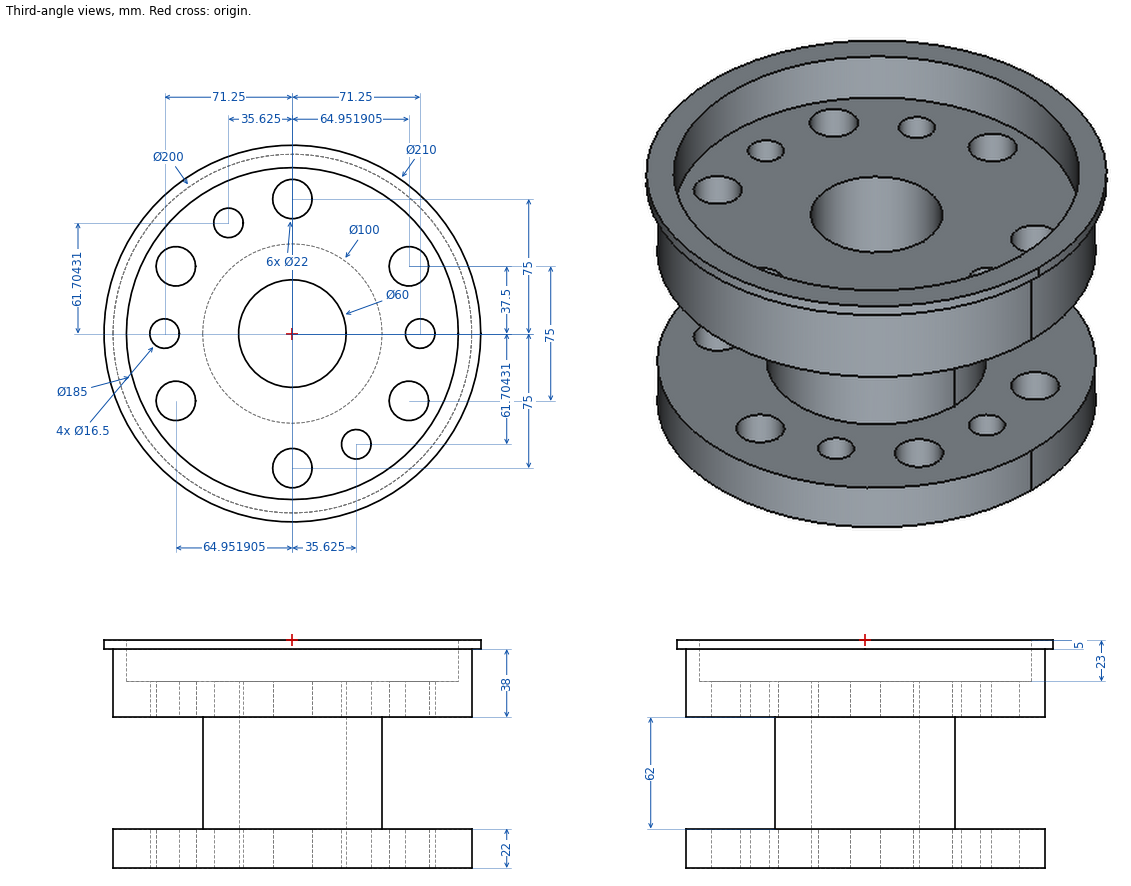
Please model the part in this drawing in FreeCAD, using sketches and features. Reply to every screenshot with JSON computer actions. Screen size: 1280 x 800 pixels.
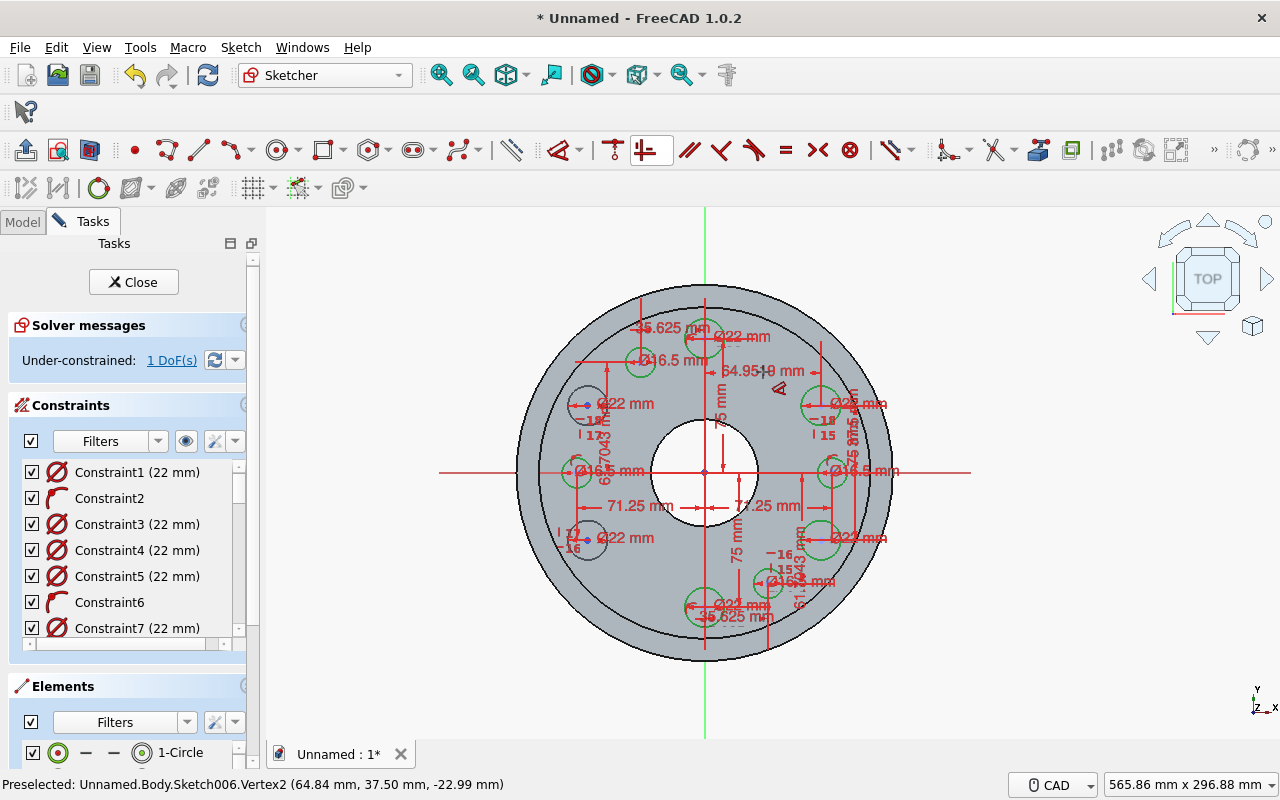
{"action": "left_click", "coordinate": [588, 540]}
{"action": "left_click", "coordinate": [646, 574]}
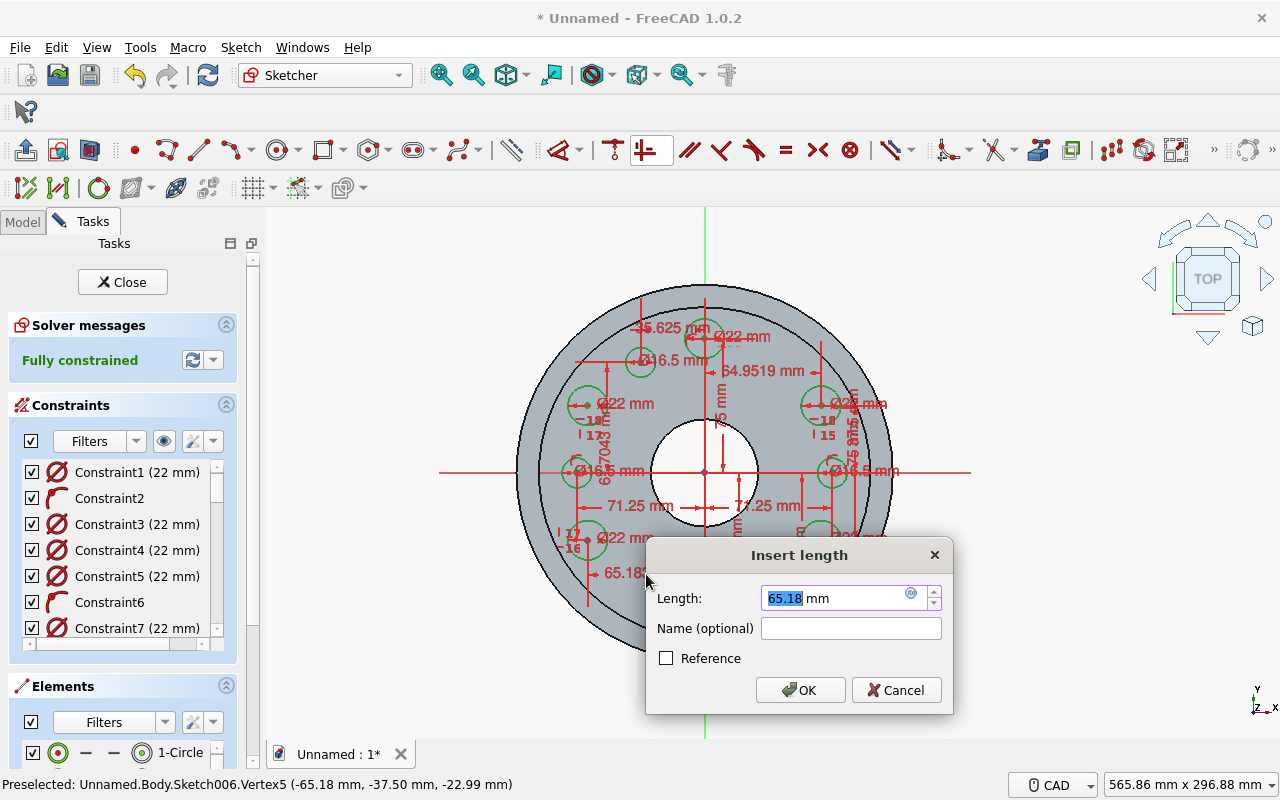
{"action": "type", "text": "64.951905"}
{"action": "key", "text": "Return"}
{"action": "key", "text": "Escape"}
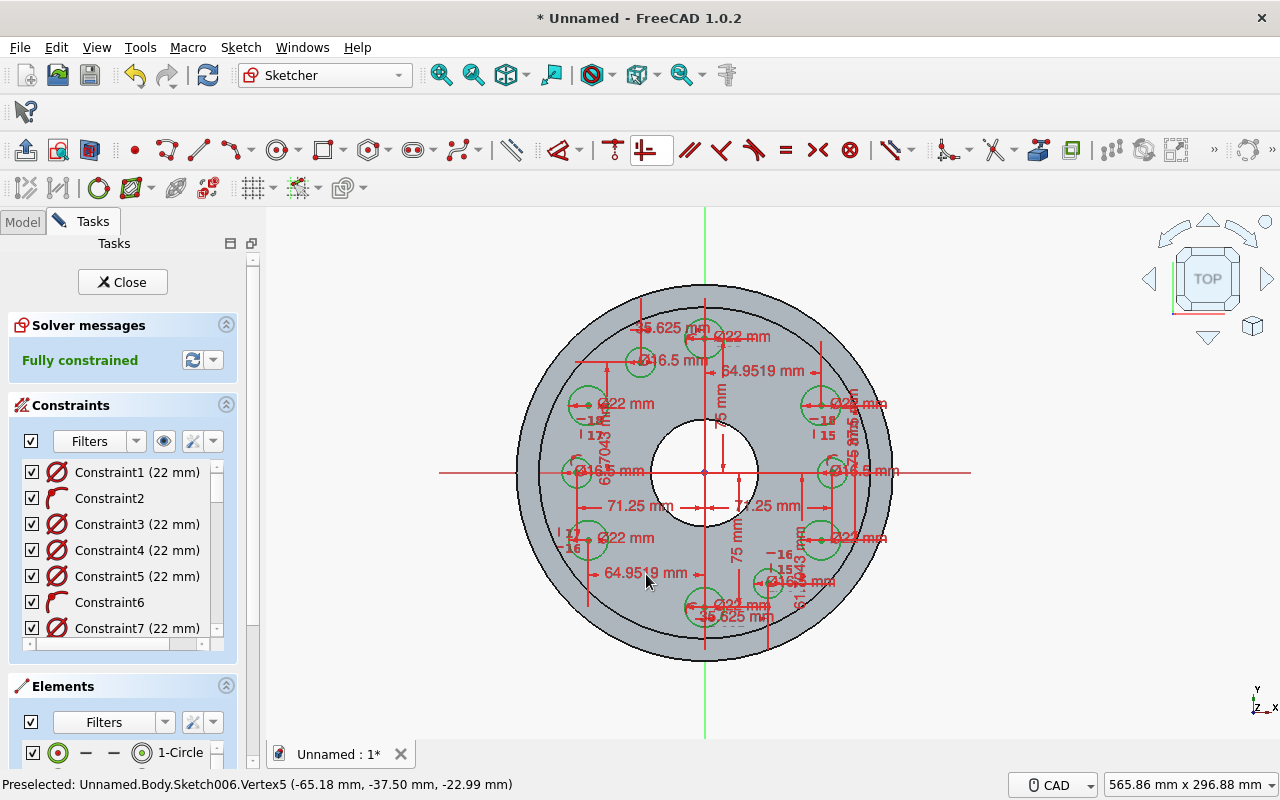
{"action": "left_click", "coordinate": [123, 282]}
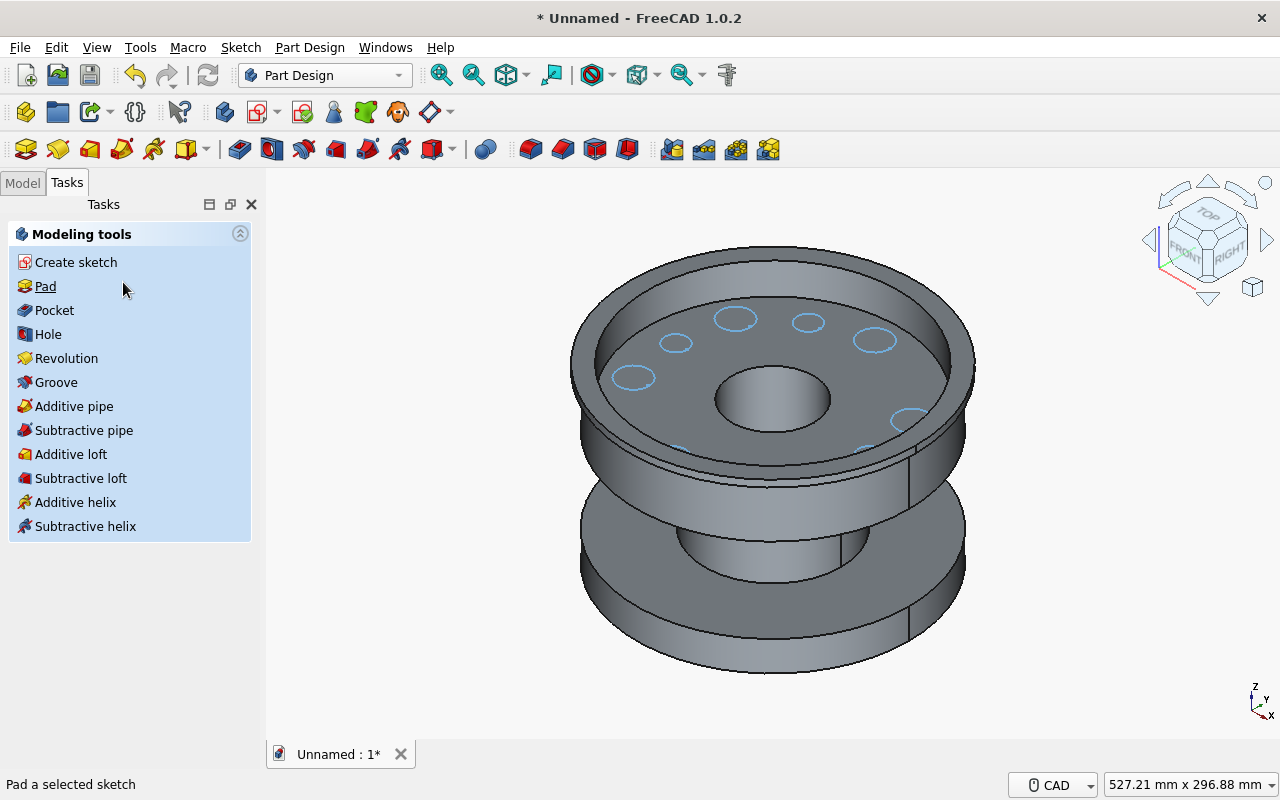
{"action": "left_click", "coordinate": [240, 150]}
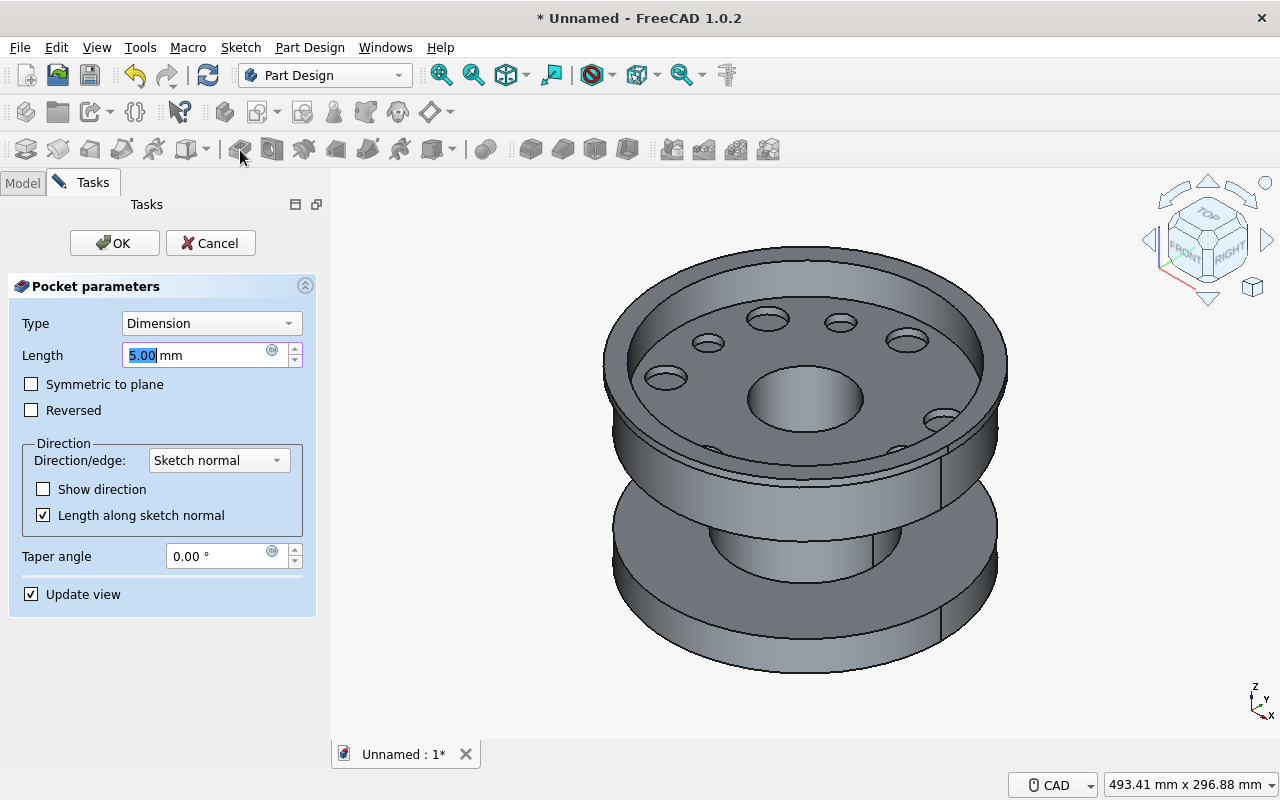
{"action": "left_click", "coordinate": [212, 324]}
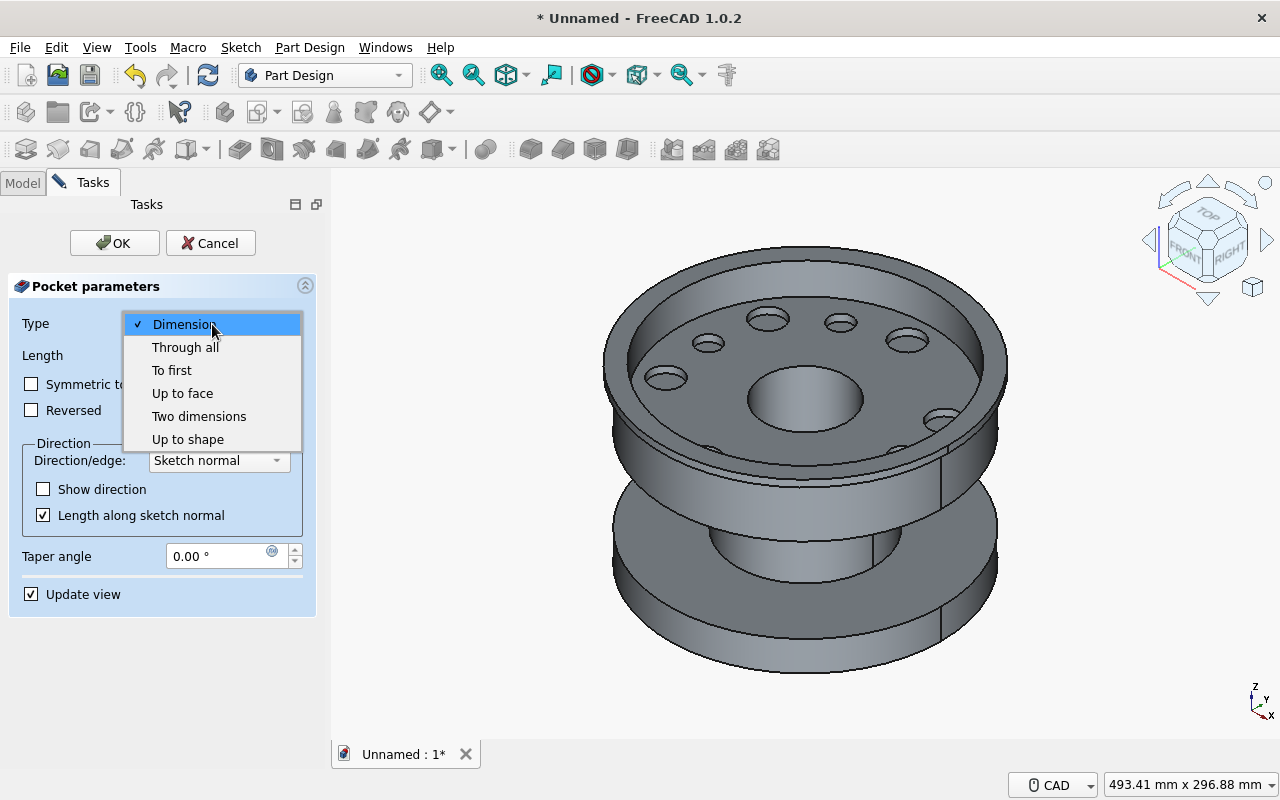
{"action": "left_click", "coordinate": [212, 348]}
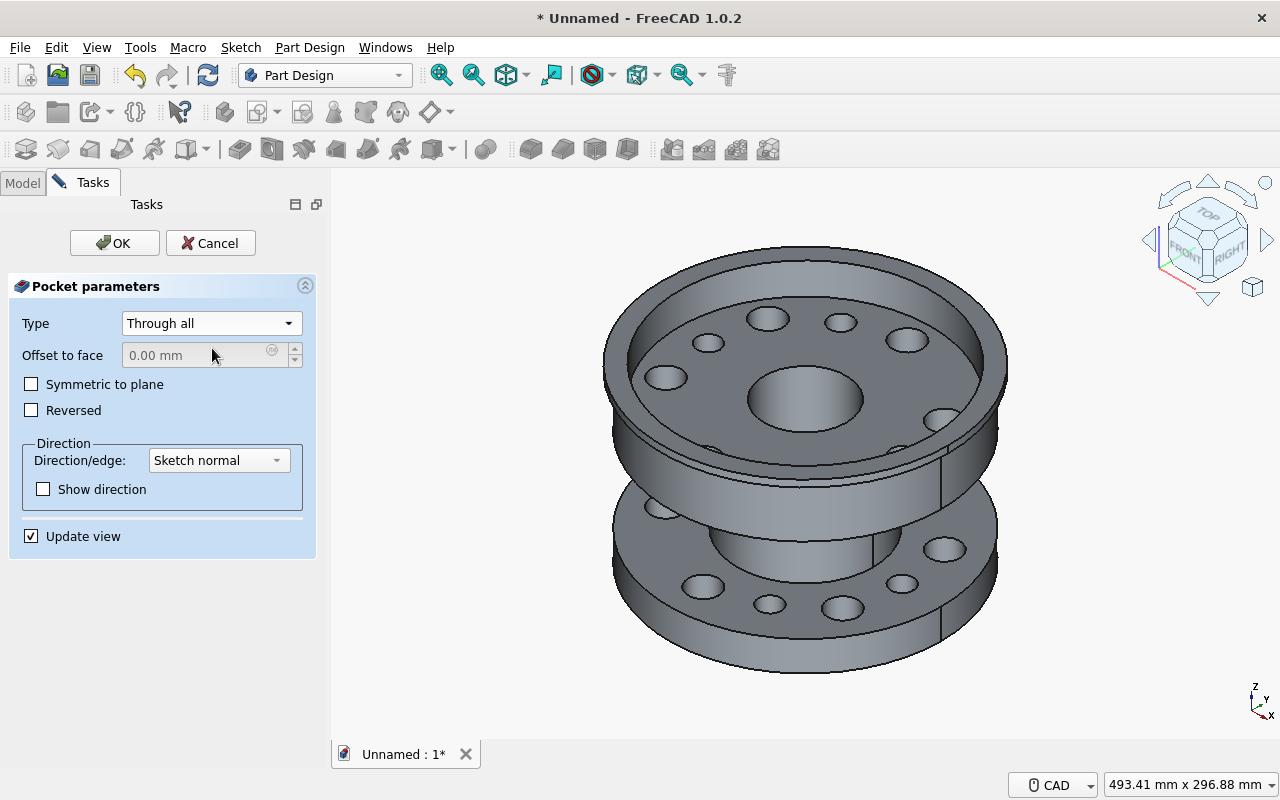
{"action": "left_click", "coordinate": [115, 243]}